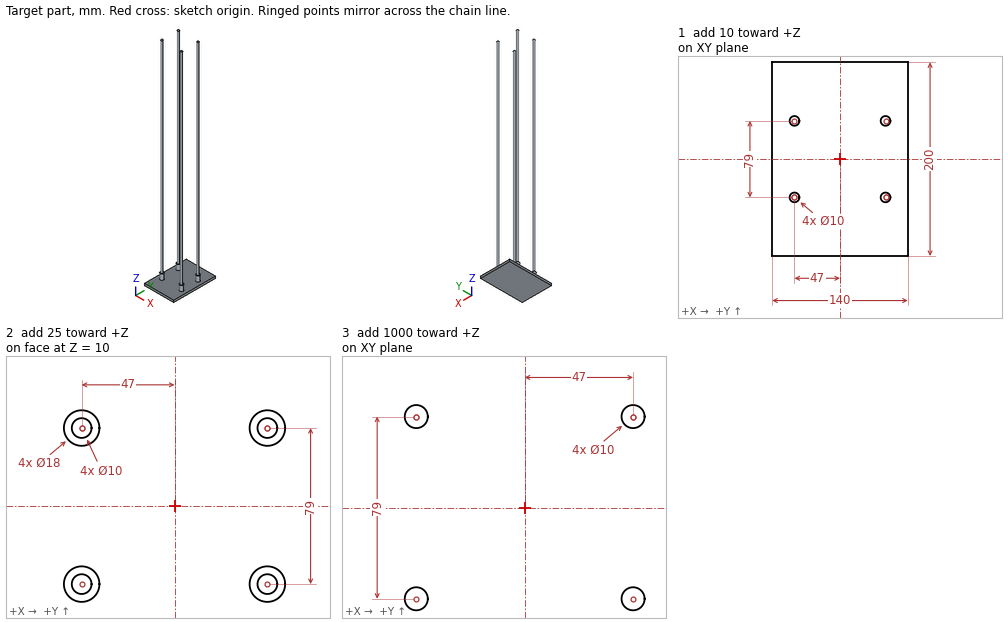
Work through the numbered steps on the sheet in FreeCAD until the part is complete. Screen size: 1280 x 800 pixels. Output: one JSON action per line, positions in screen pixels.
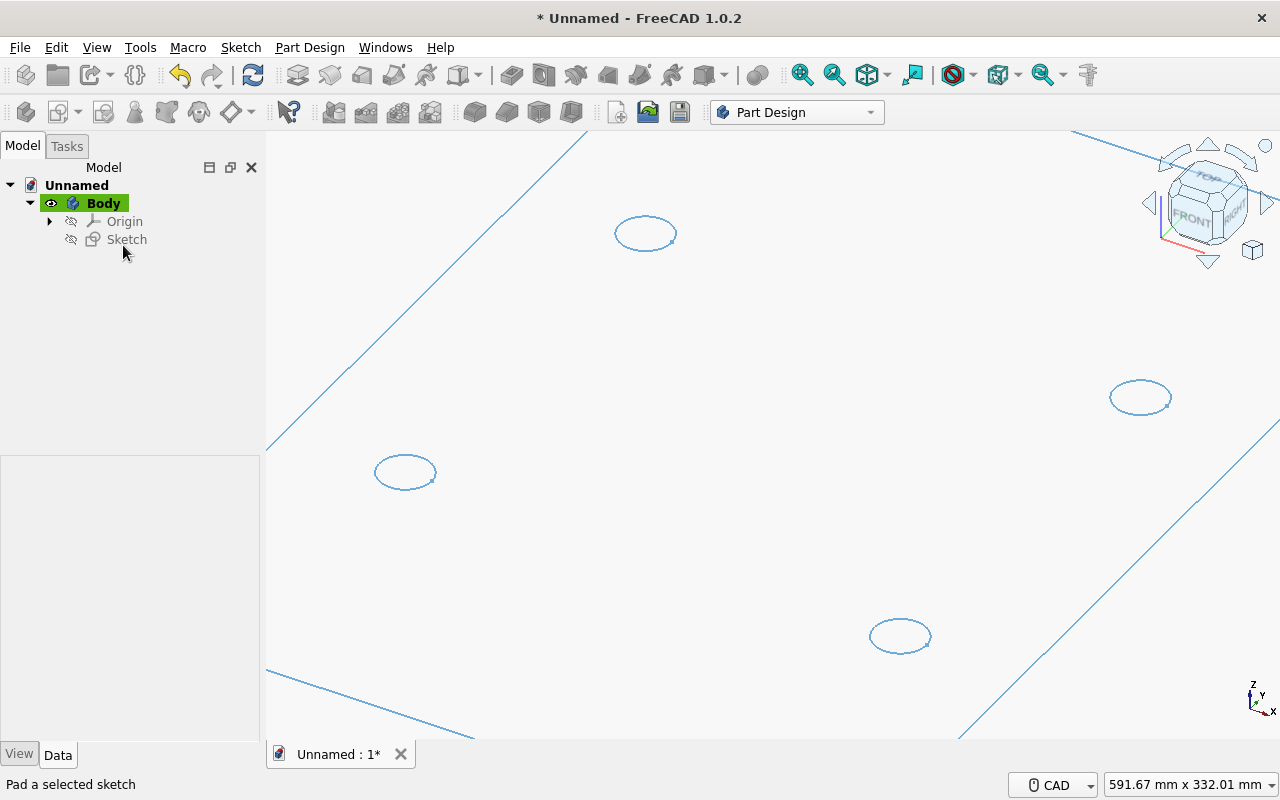
{"action": "left_click", "coordinate": [298, 76]}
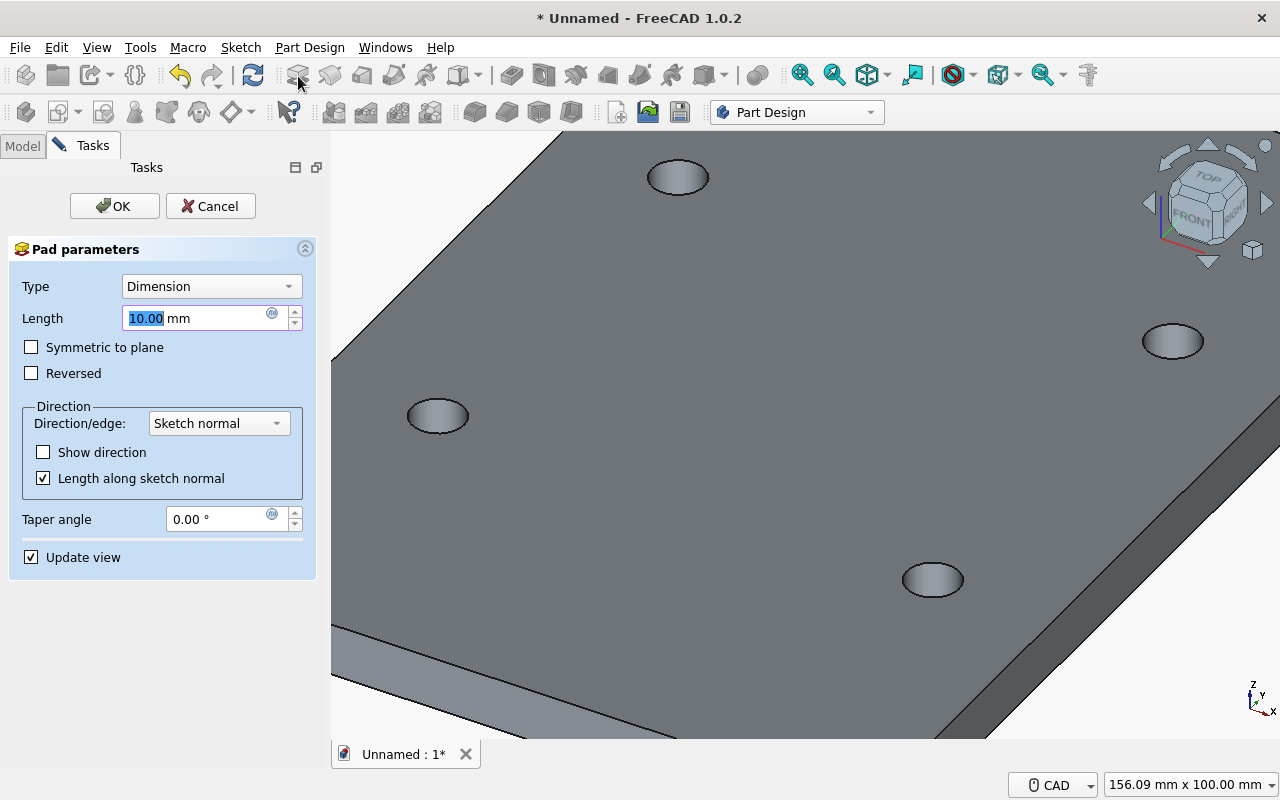
{"action": "type", "text": "10"}
{"action": "key", "text": "Tab"}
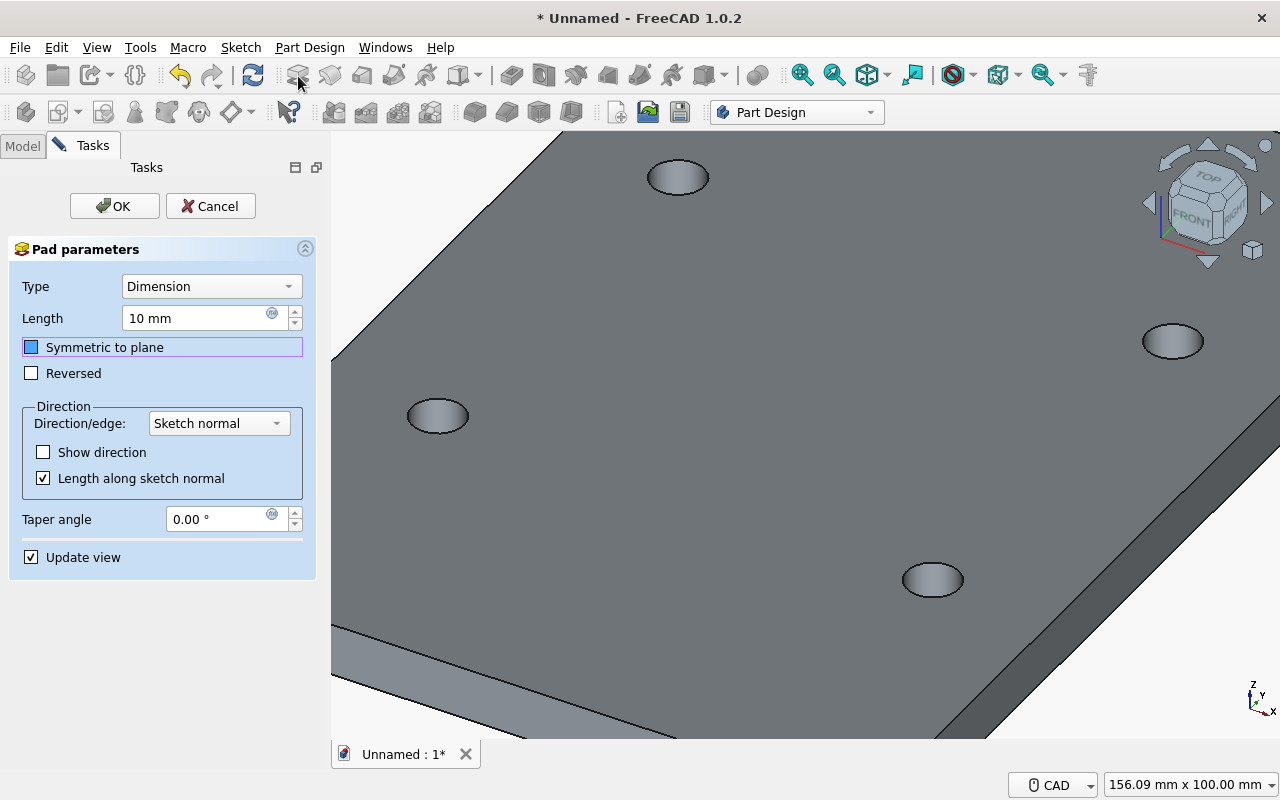
{"action": "left_click", "coordinate": [115, 206]}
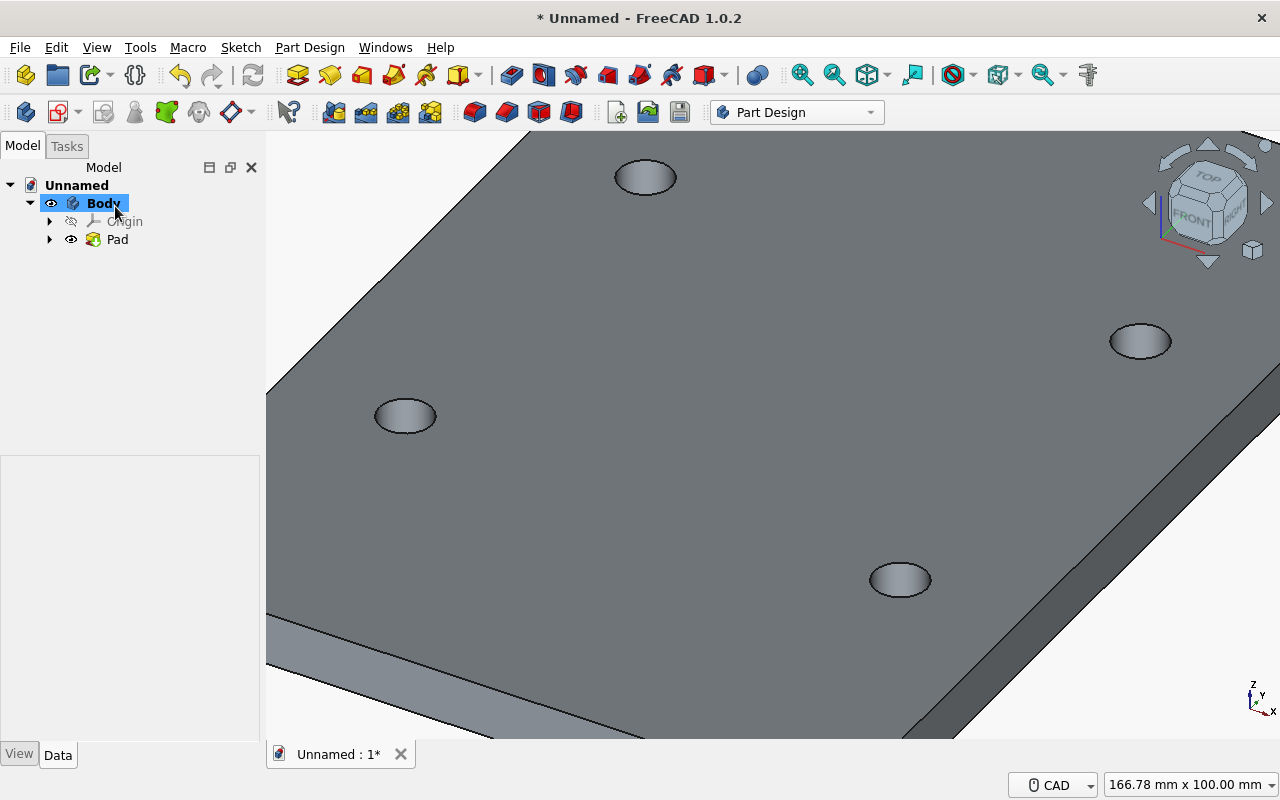
{"action": "left_click", "coordinate": [804, 76]}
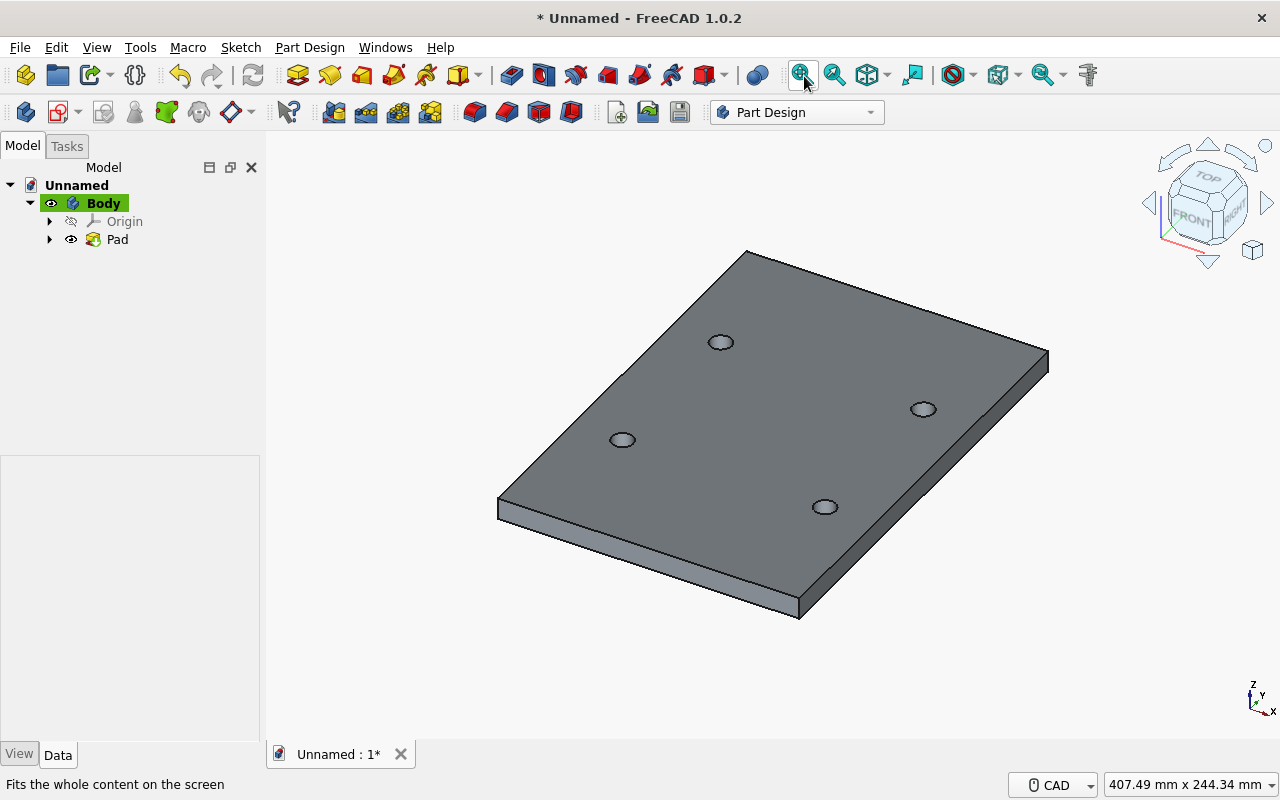
{"action": "left_click", "coordinate": [773, 424]}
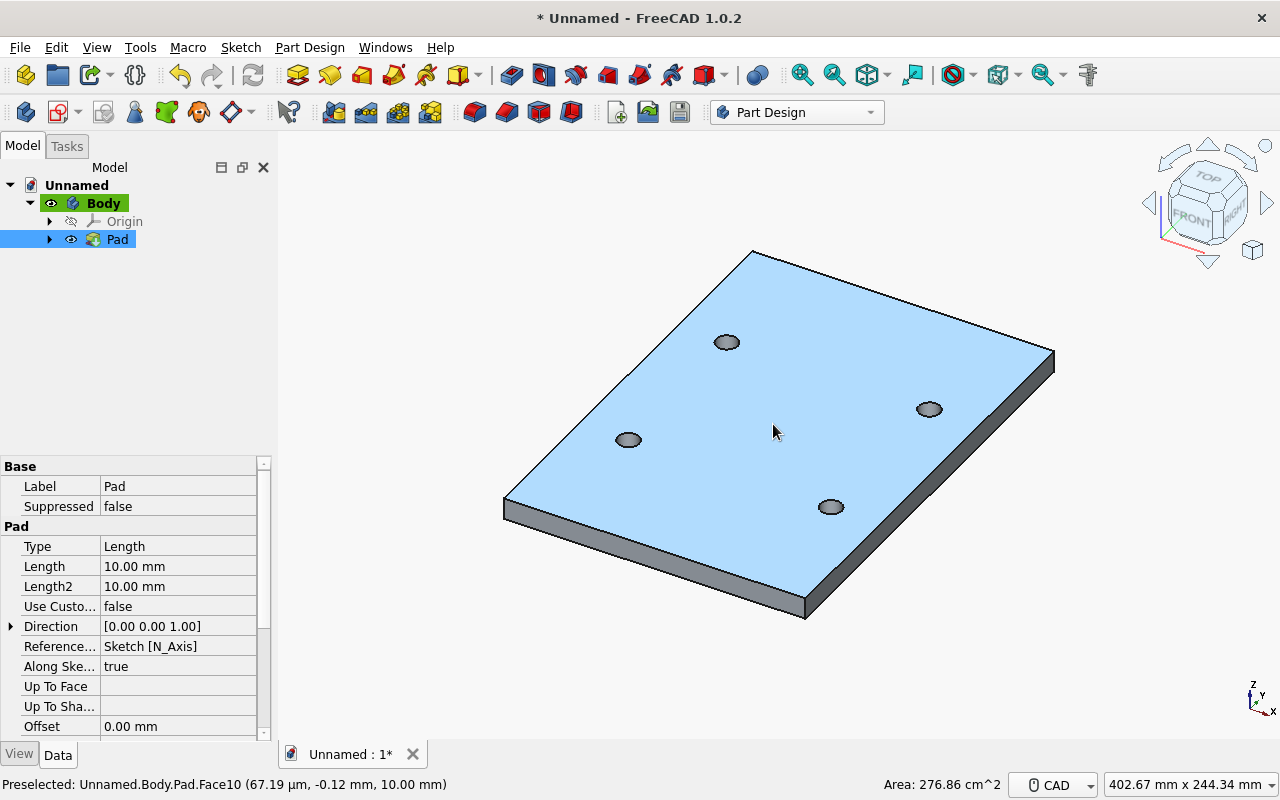
{"action": "left_click", "coordinate": [58, 112]}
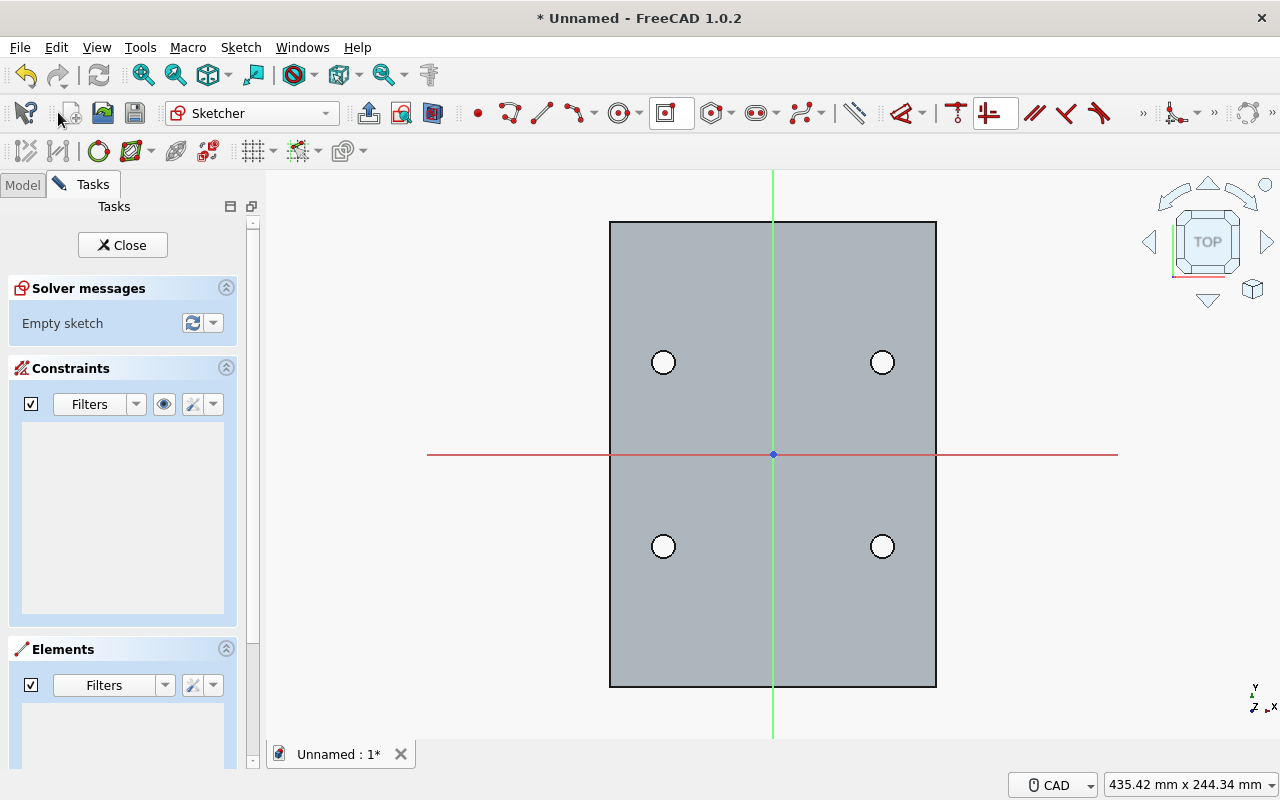
{"action": "scroll", "coordinate": [912, 455], "scroll_direction": "up", "scroll_amount": 2}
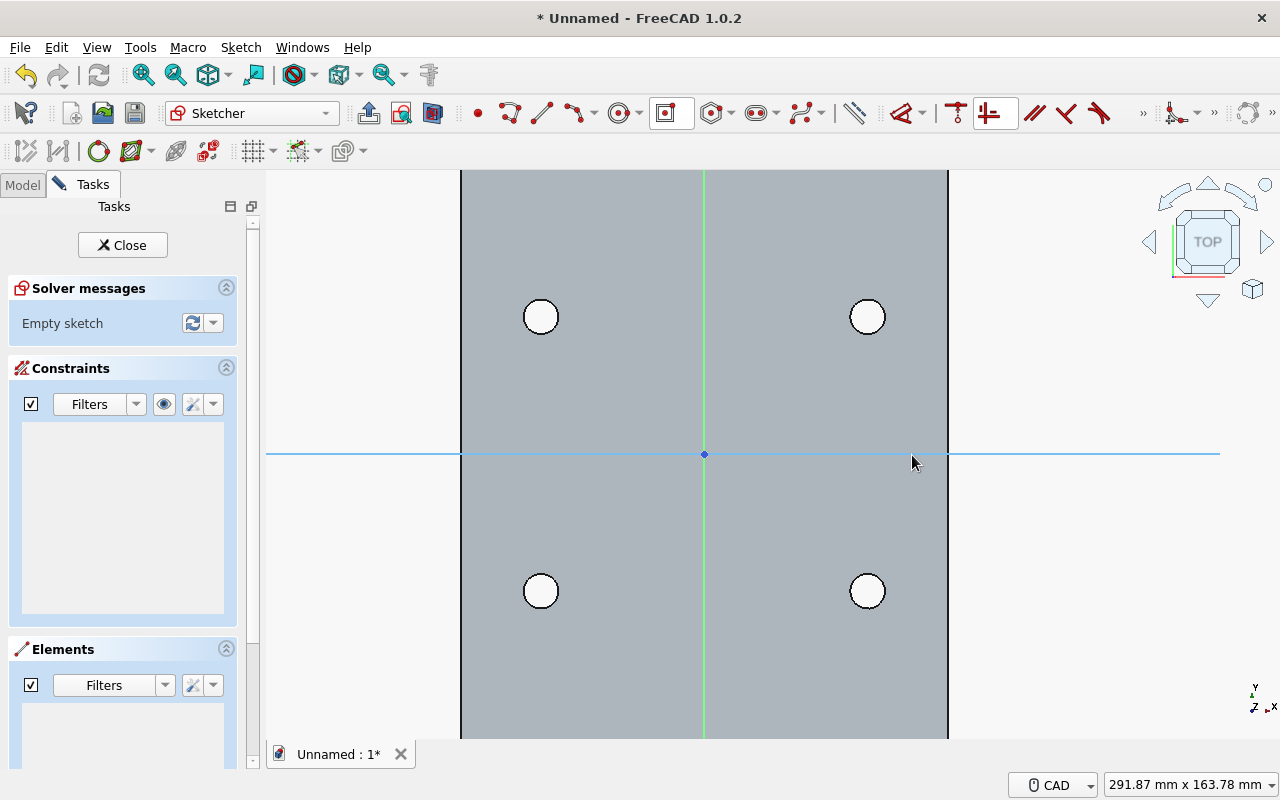
{"action": "left_click", "coordinate": [620, 114]}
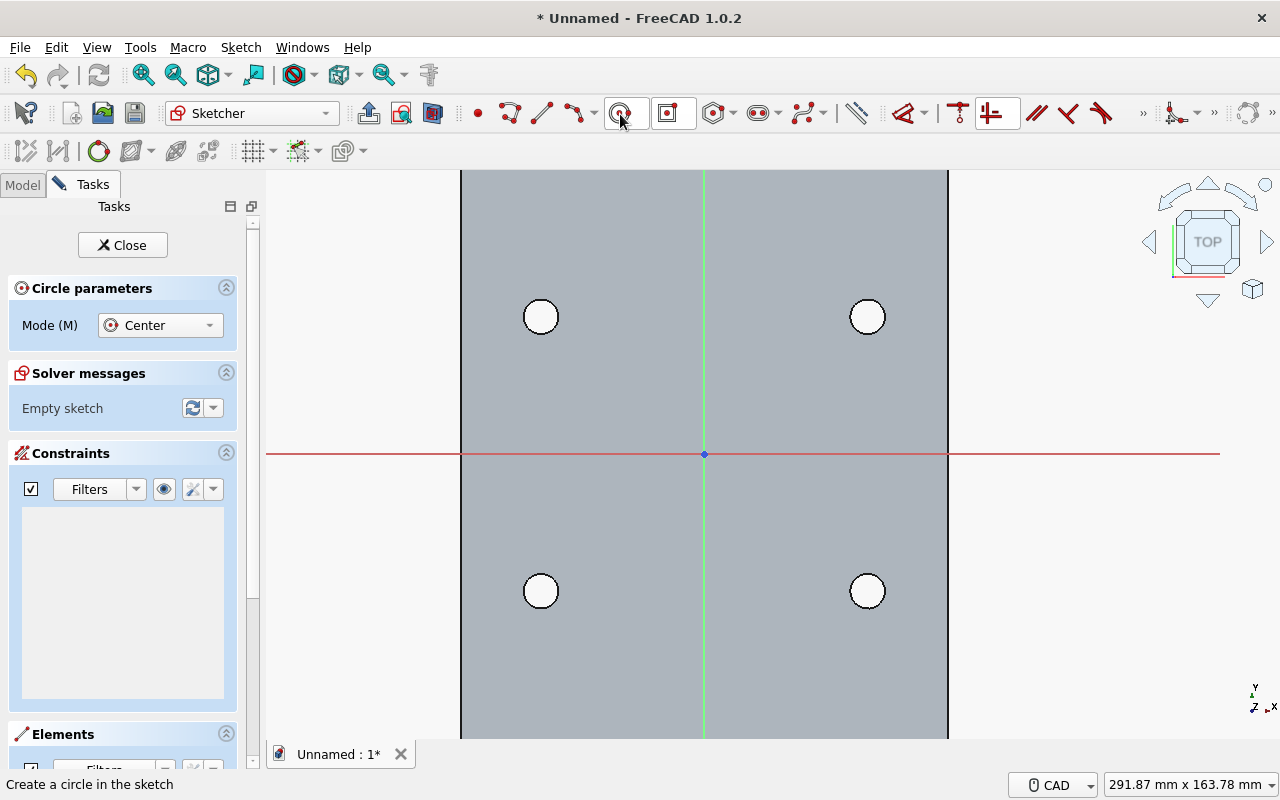
{"action": "left_click", "coordinate": [541, 317]}
{"action": "left_click", "coordinate": [563, 295]}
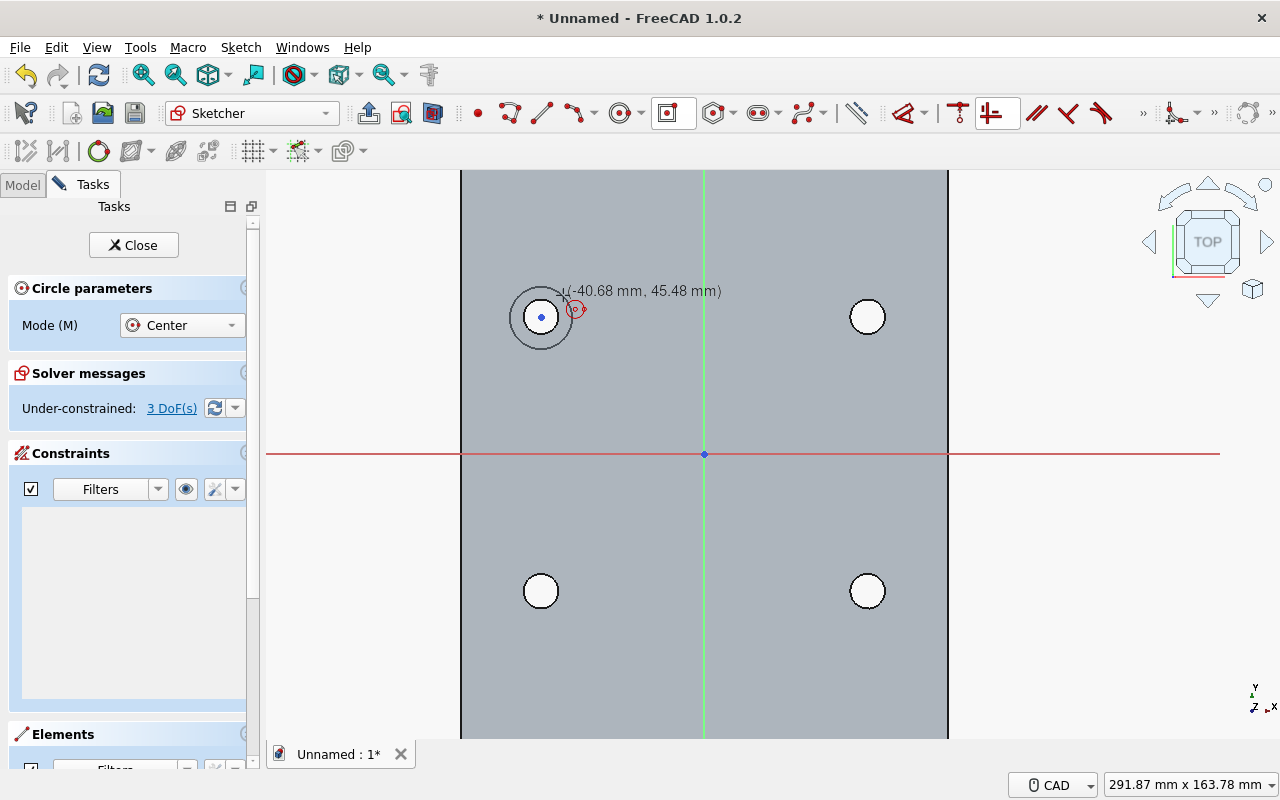
{"action": "left_click", "coordinate": [868, 317]}
{"action": "left_click", "coordinate": [890, 295]}